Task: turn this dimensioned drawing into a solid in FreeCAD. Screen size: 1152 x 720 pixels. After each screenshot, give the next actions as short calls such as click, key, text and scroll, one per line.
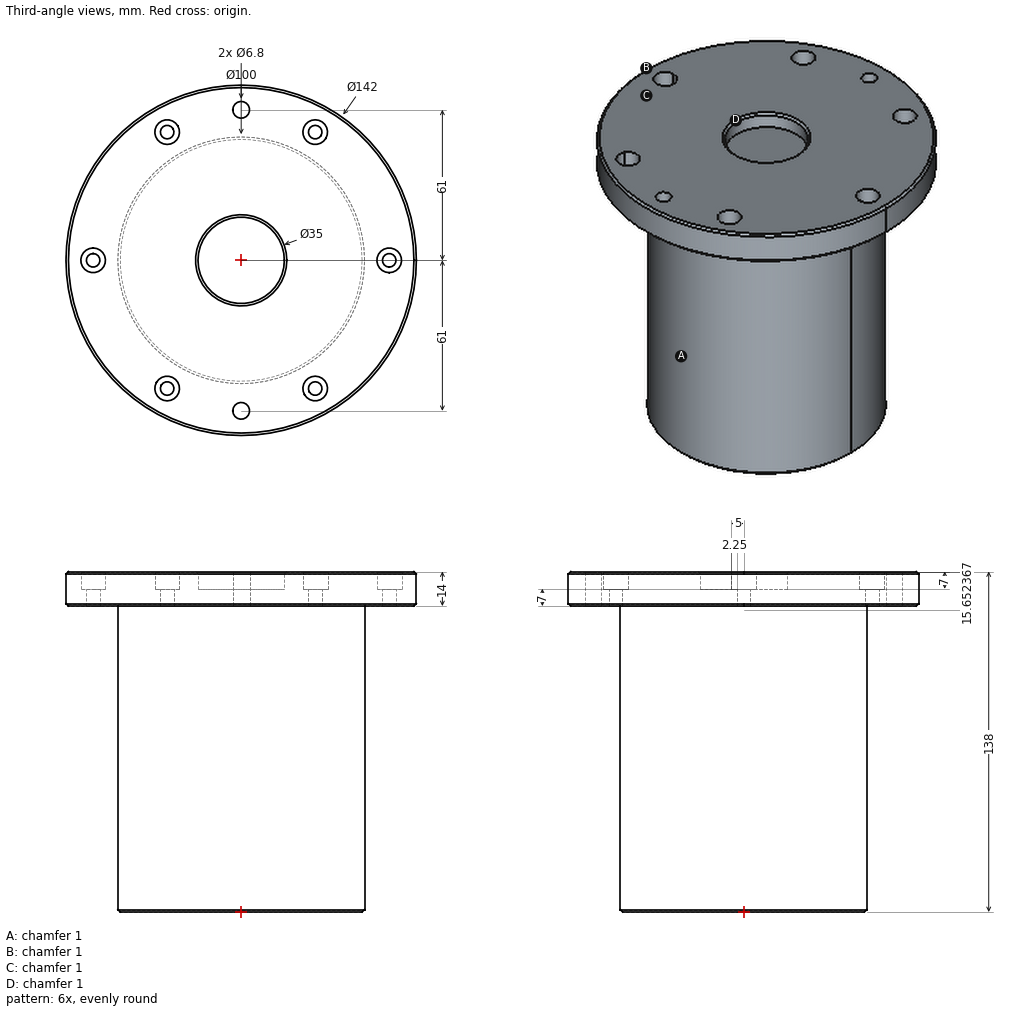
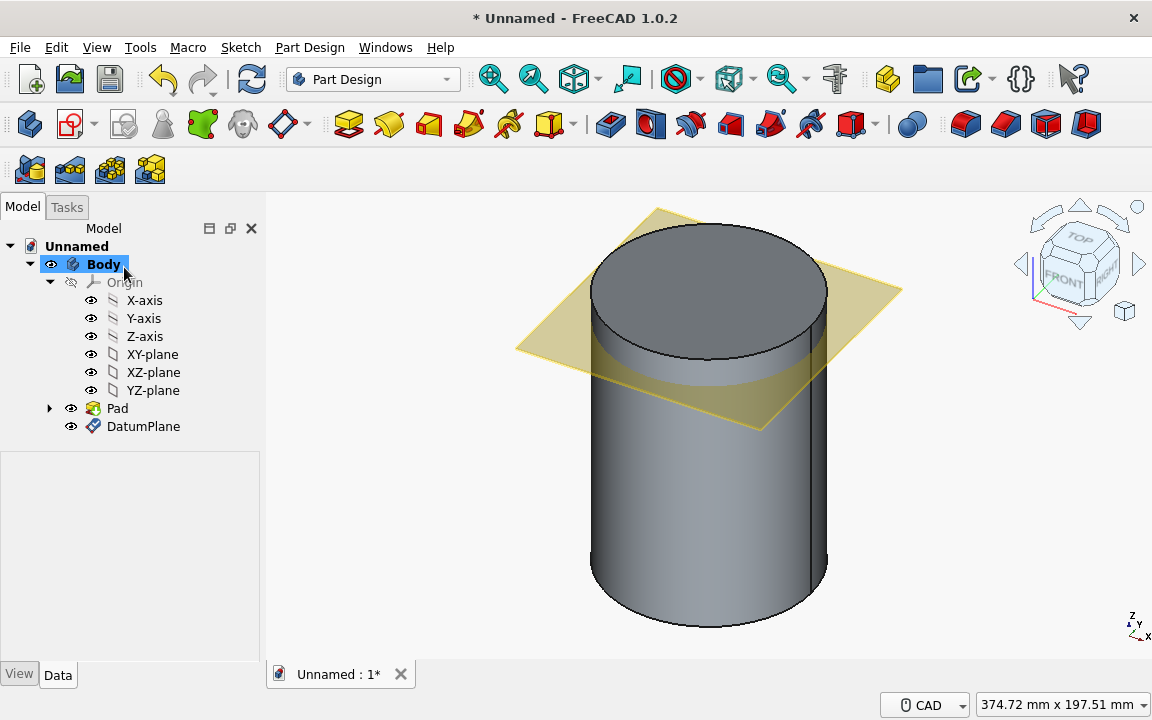
click(116, 426)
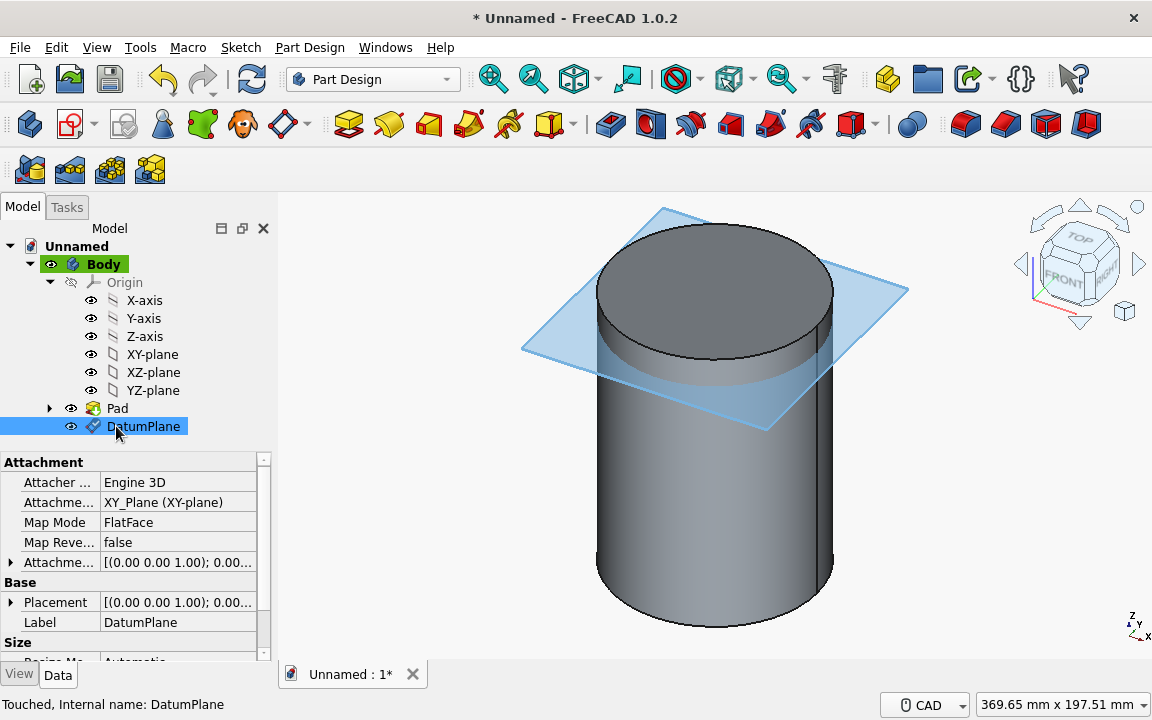
click(70, 124)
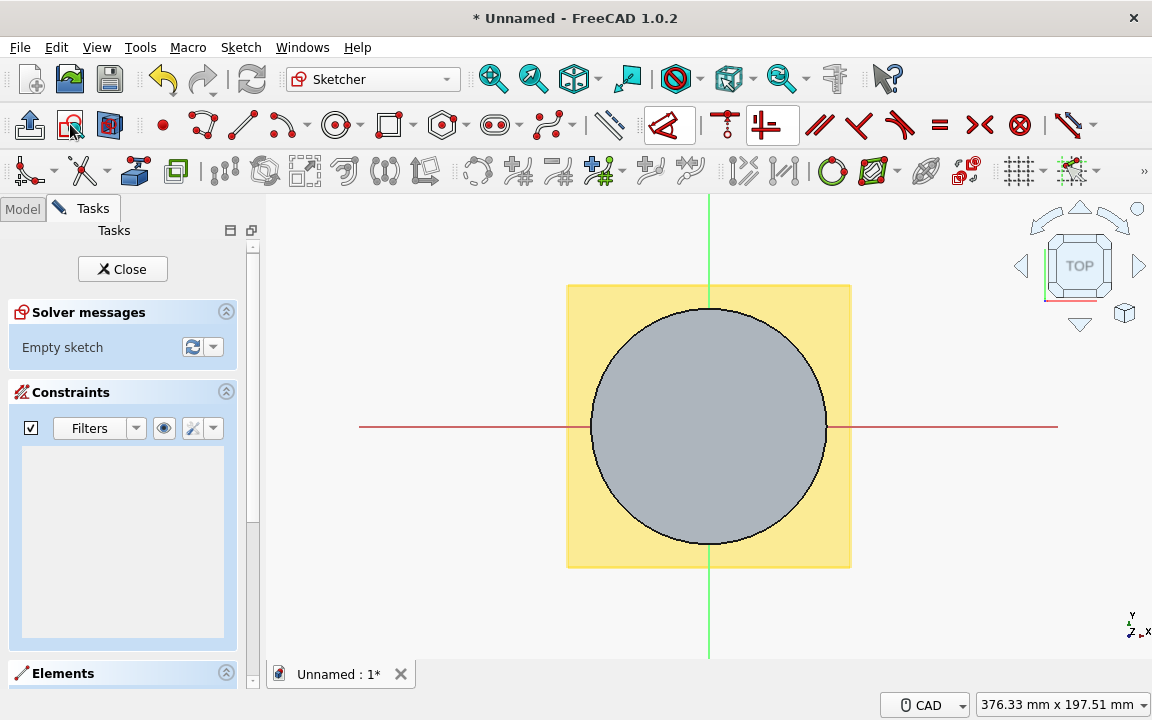
key(q)
key(s)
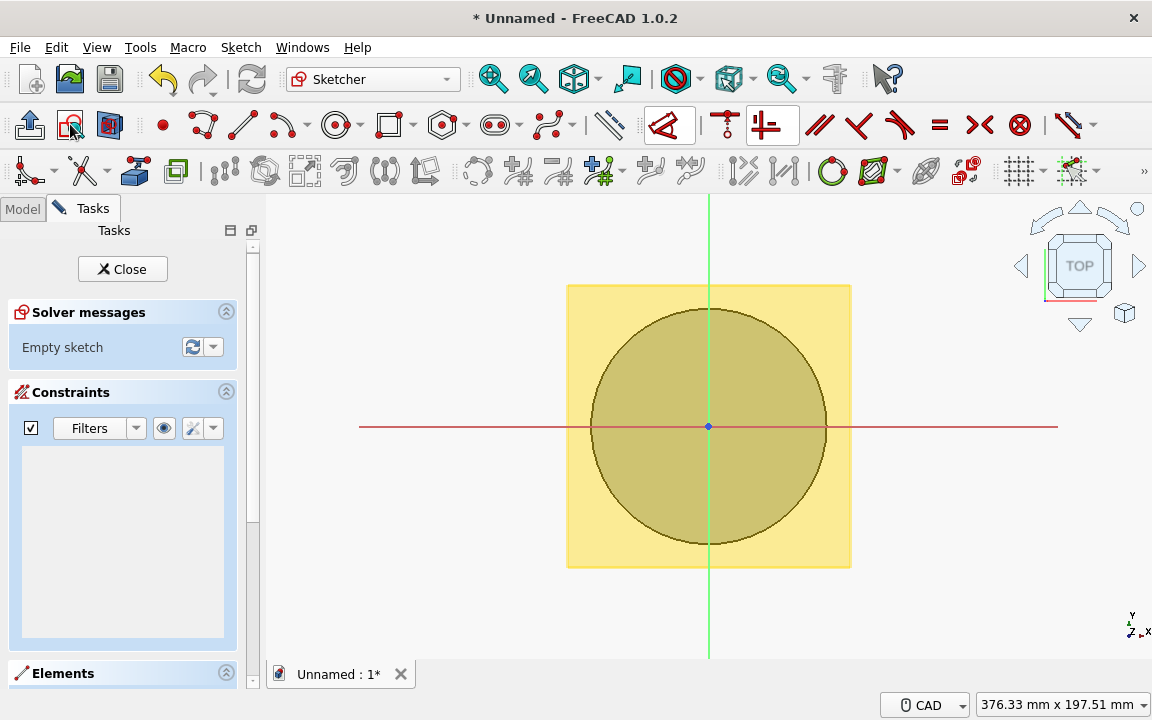
click(336, 126)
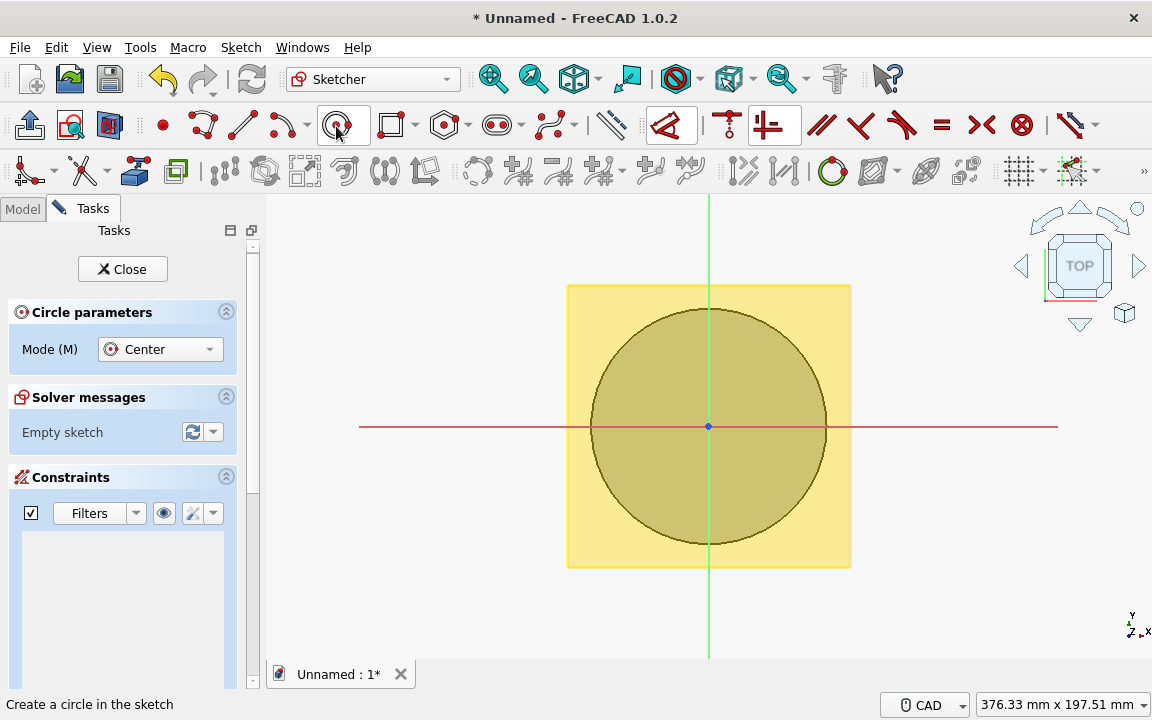
click(709, 426)
click(827, 308)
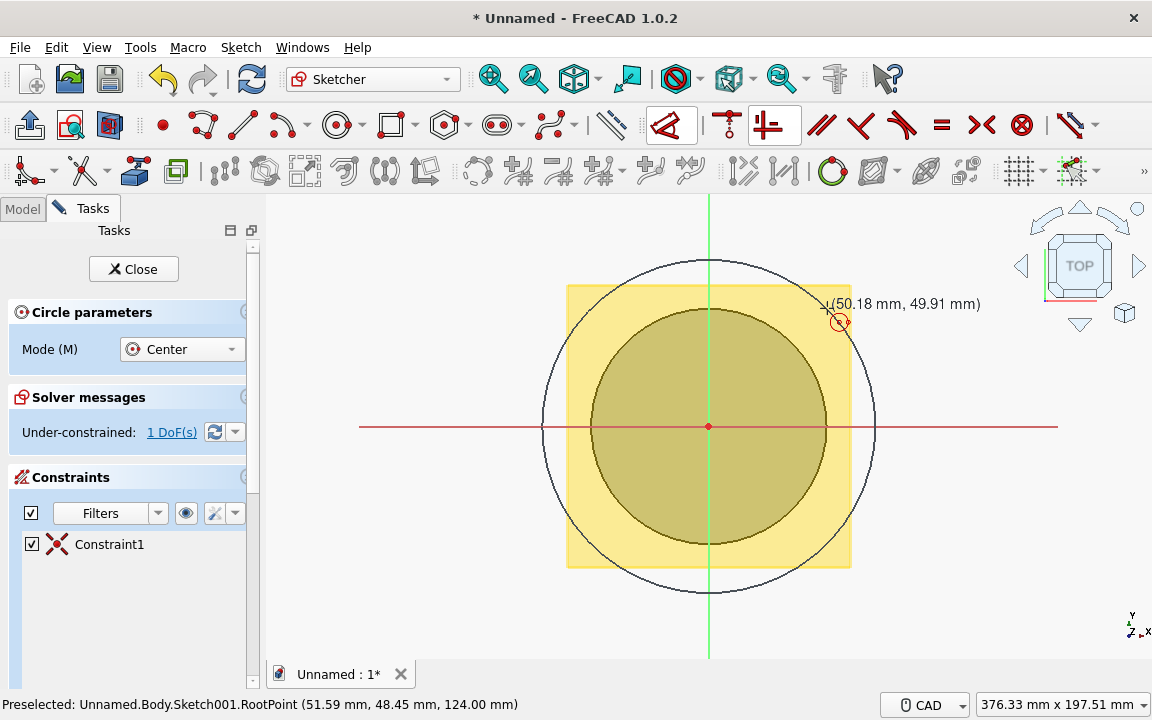
click(709, 426)
click(792, 343)
key(Escape)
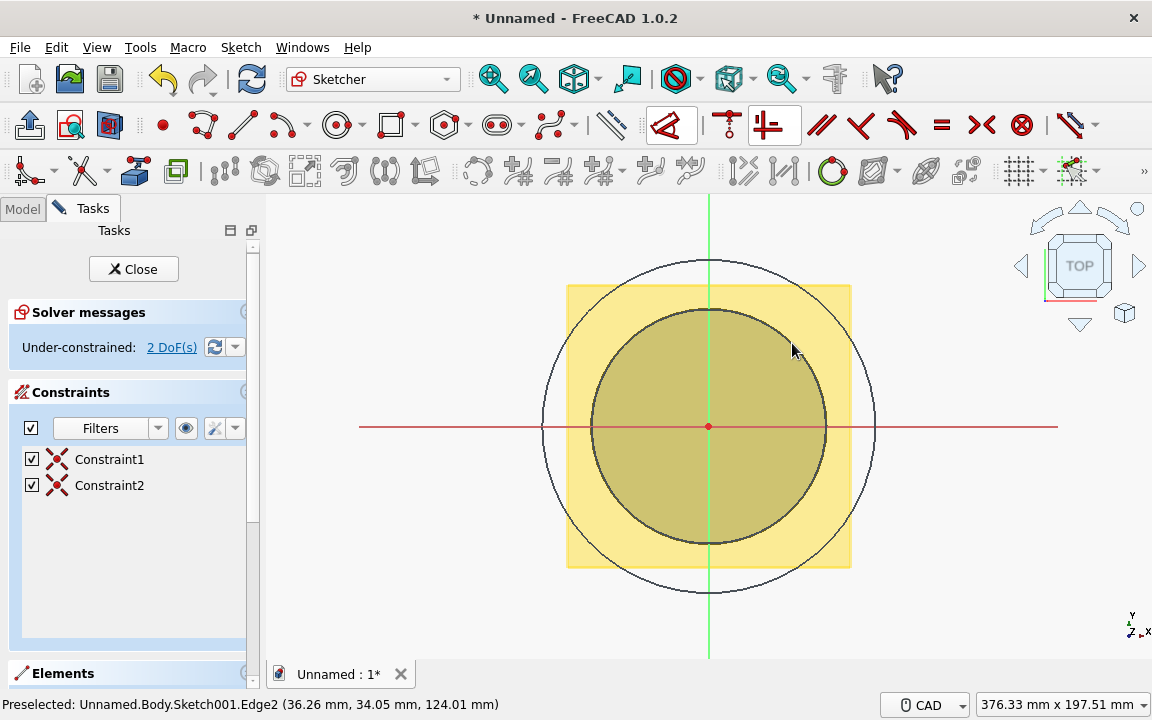
click(826, 308)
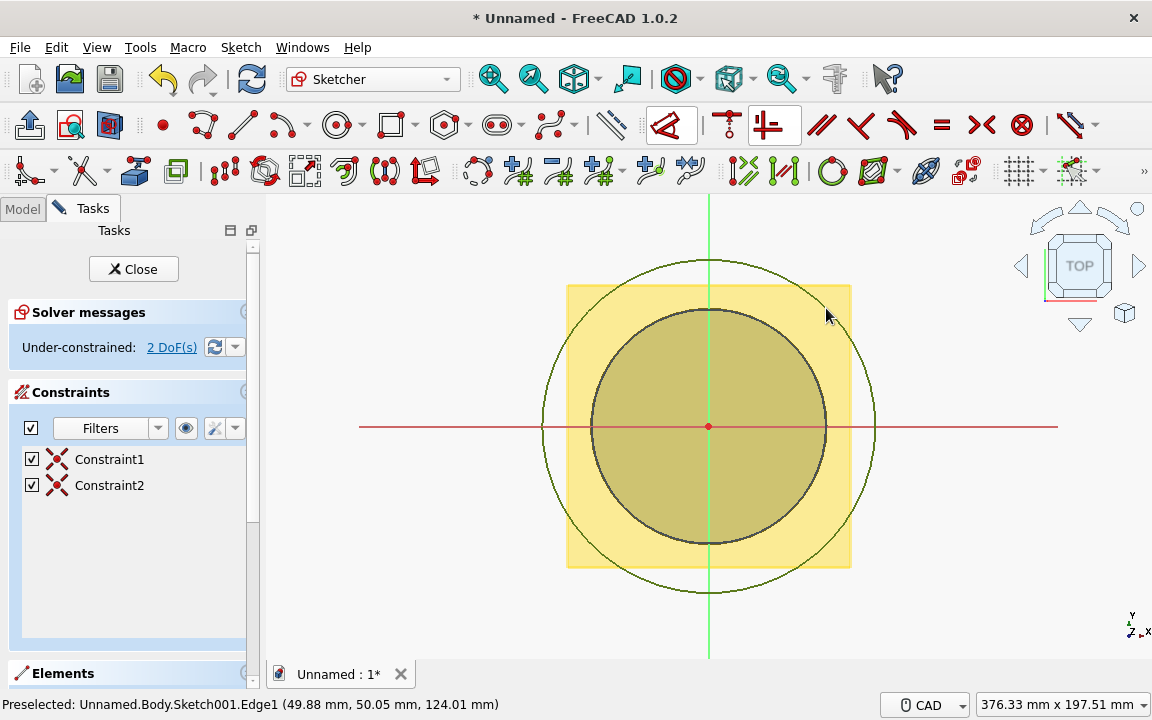
key(k)
key(o)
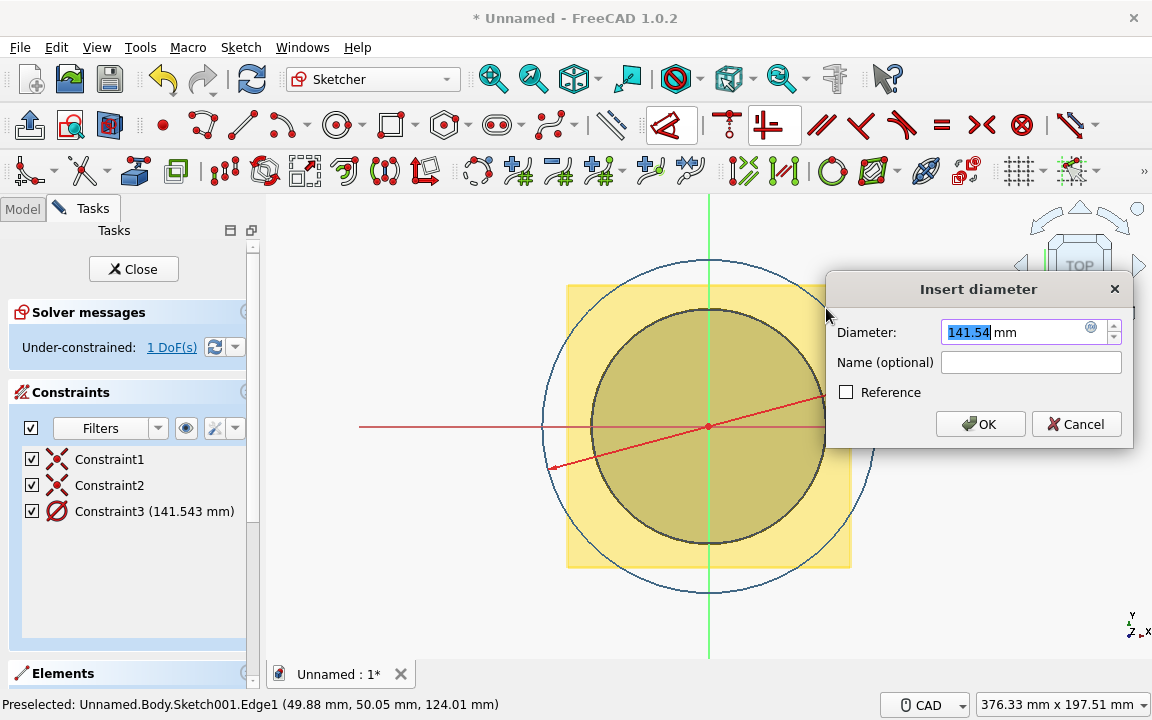
text(142)
key(Return)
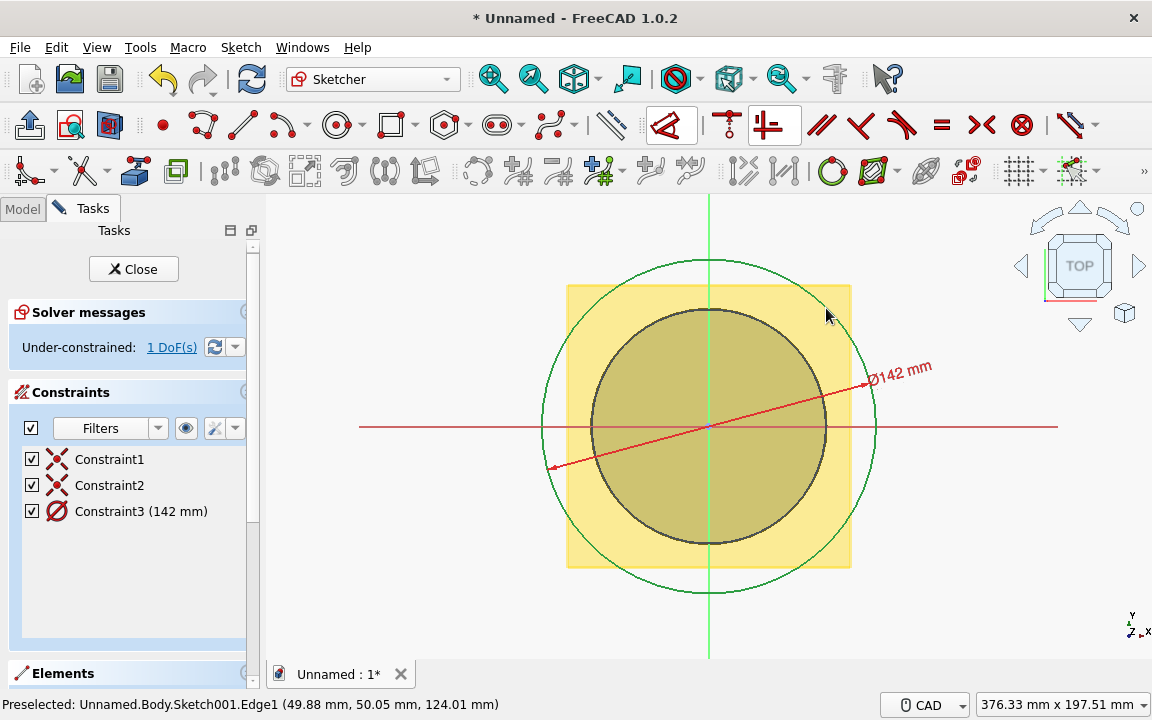
click(791, 343)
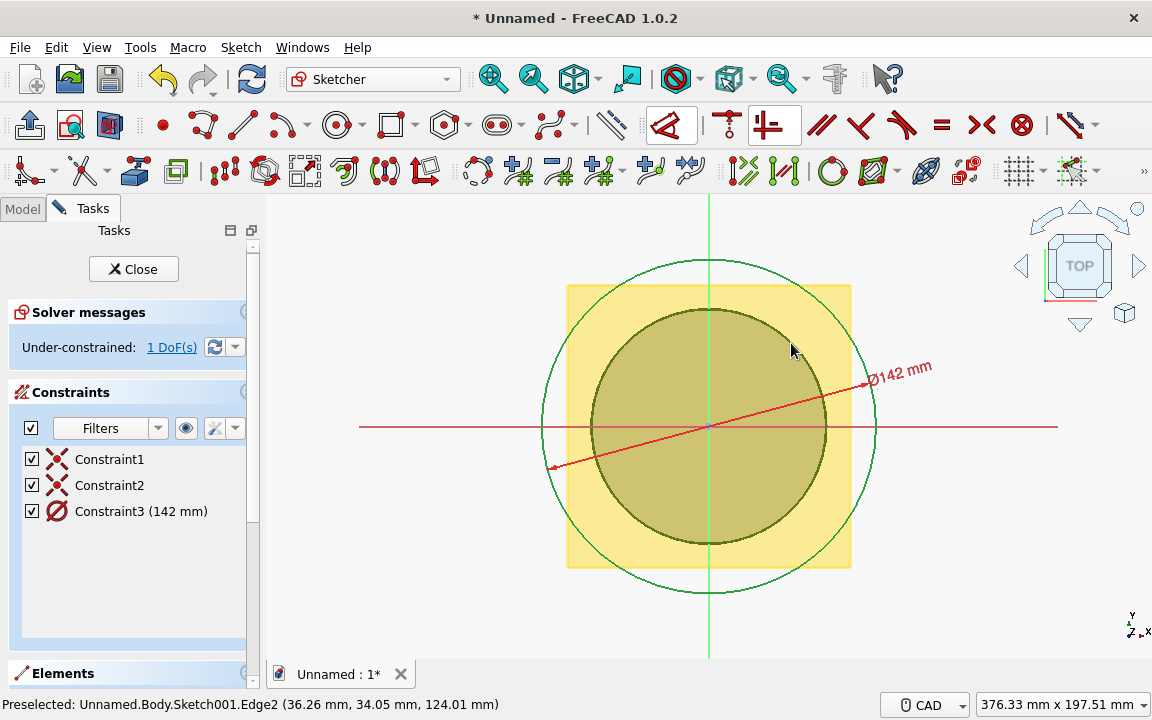
key(k)
key(o)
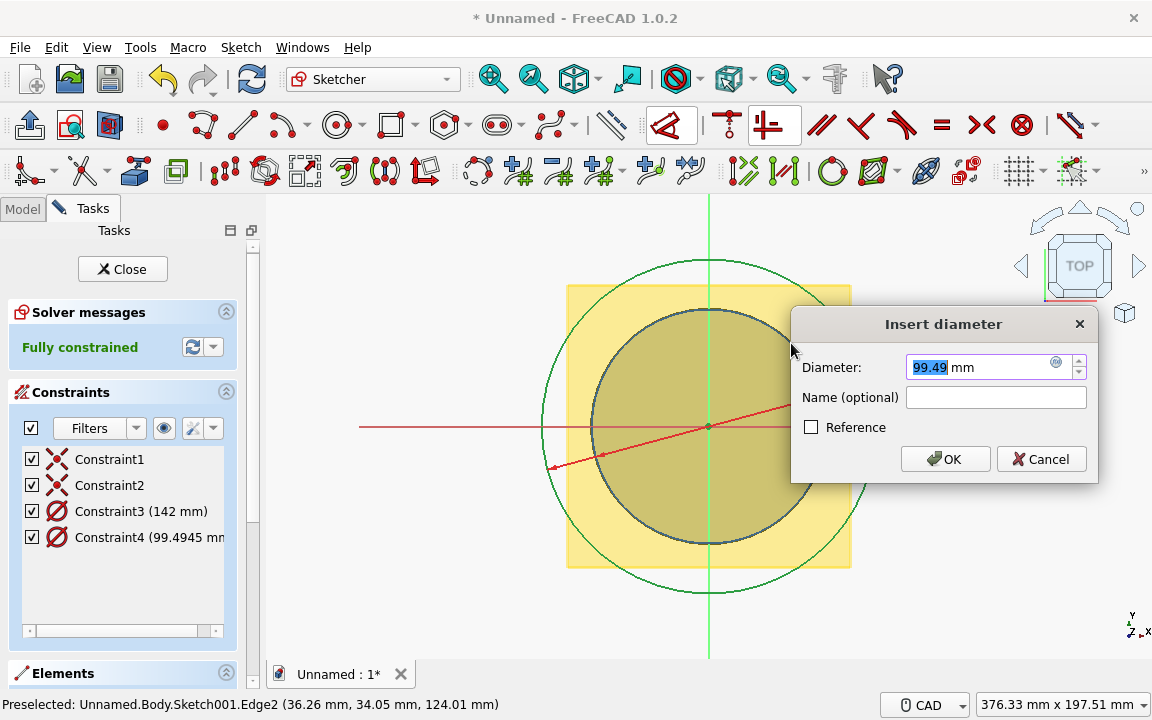
text(100)
key(Return)